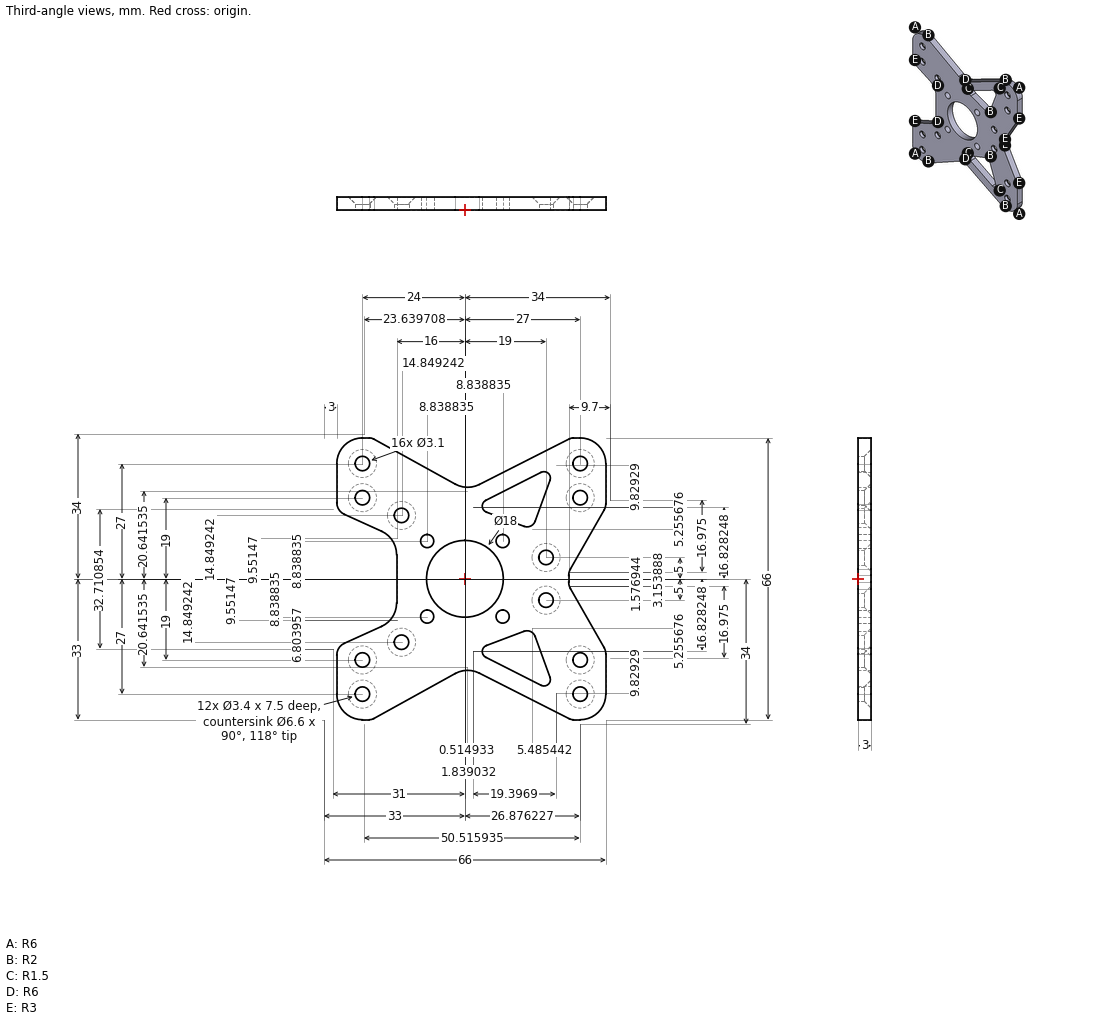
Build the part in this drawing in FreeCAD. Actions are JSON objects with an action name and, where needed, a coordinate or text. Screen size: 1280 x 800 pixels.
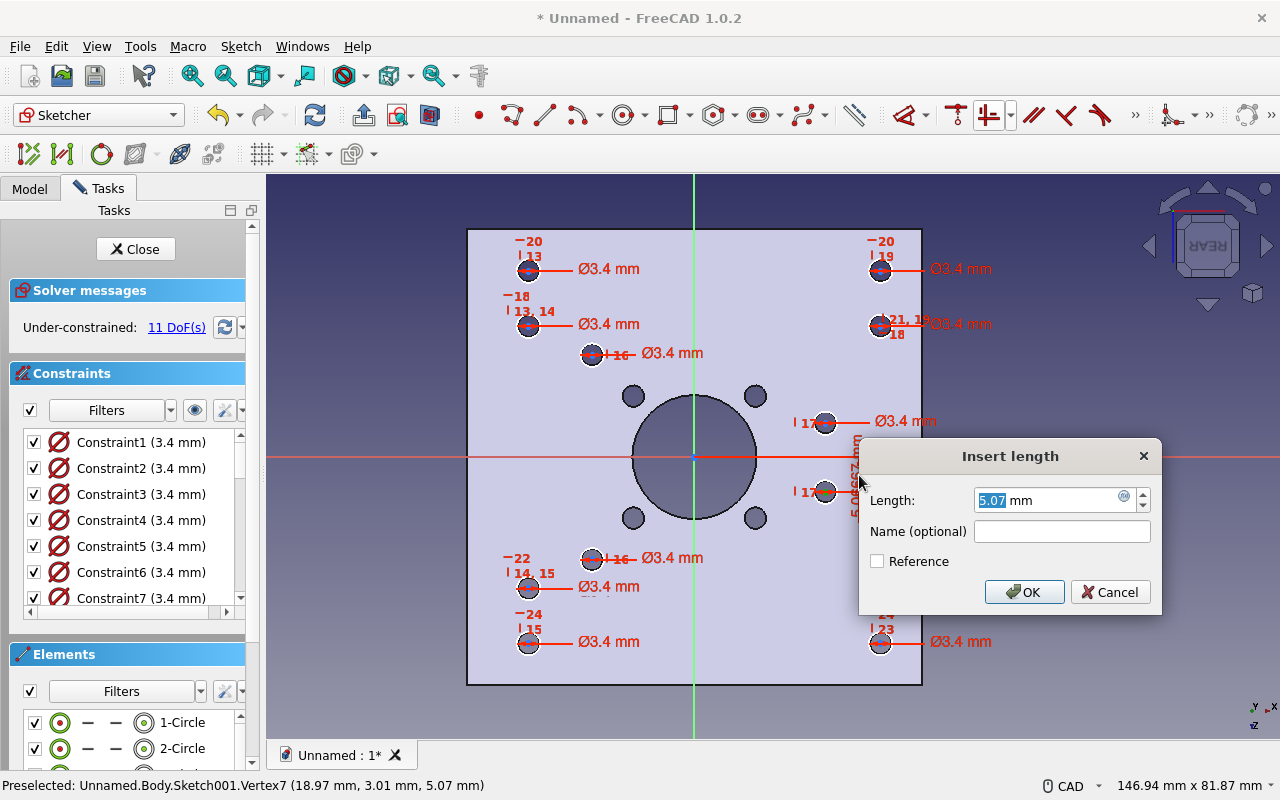
{"action": "type", "text": "5"}
{"action": "key", "text": "Return"}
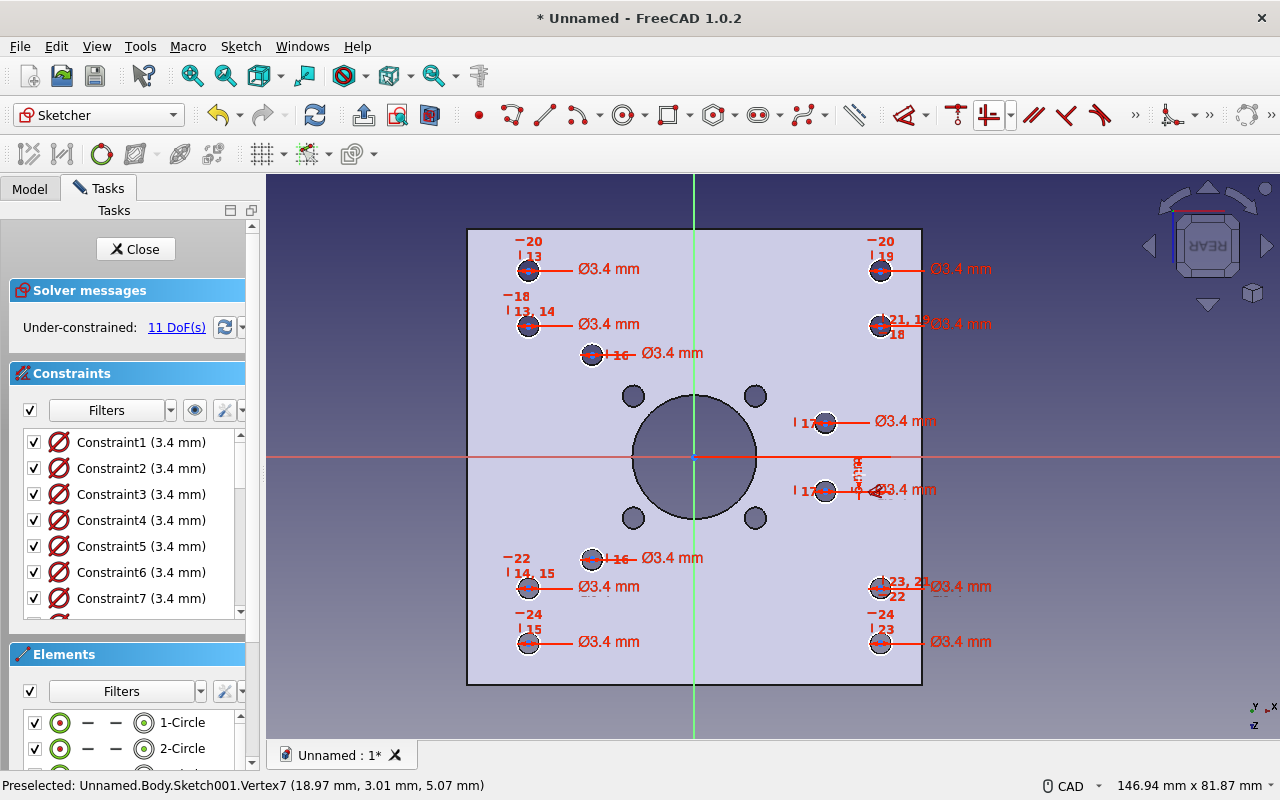
{"action": "left_click", "coordinate": [825, 423]}
{"action": "left_click", "coordinate": [859, 440]}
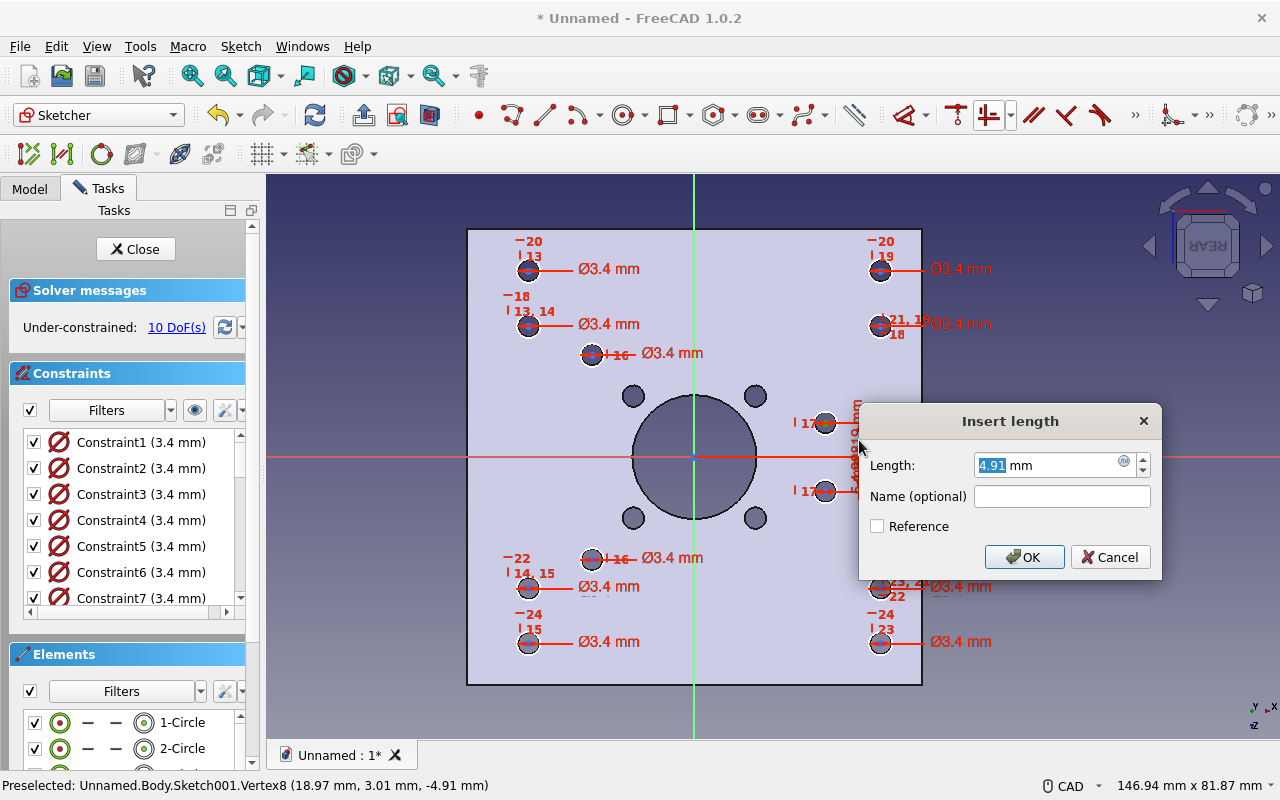
{"action": "type", "text": "5"}
{"action": "key", "text": "Return"}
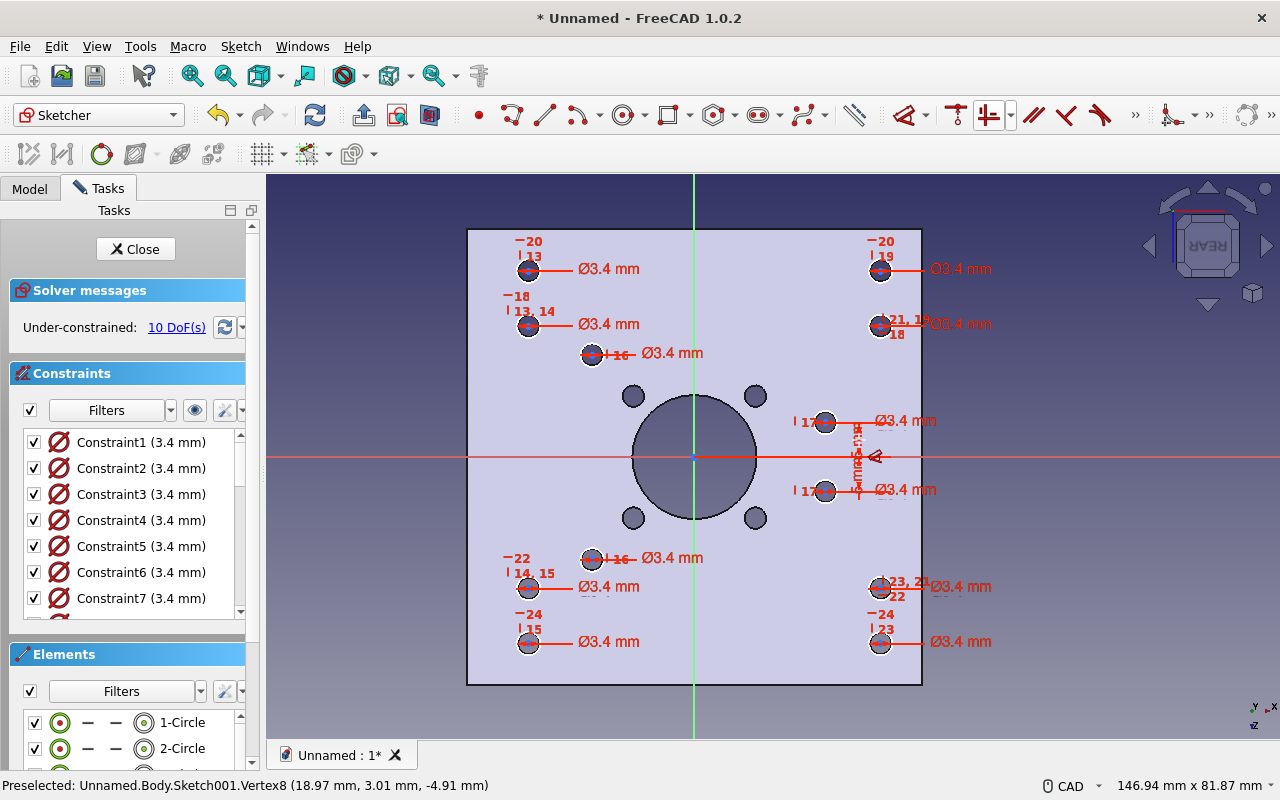
{"action": "left_click", "coordinate": [529, 271]}
{"action": "left_click", "coordinate": [612, 237]}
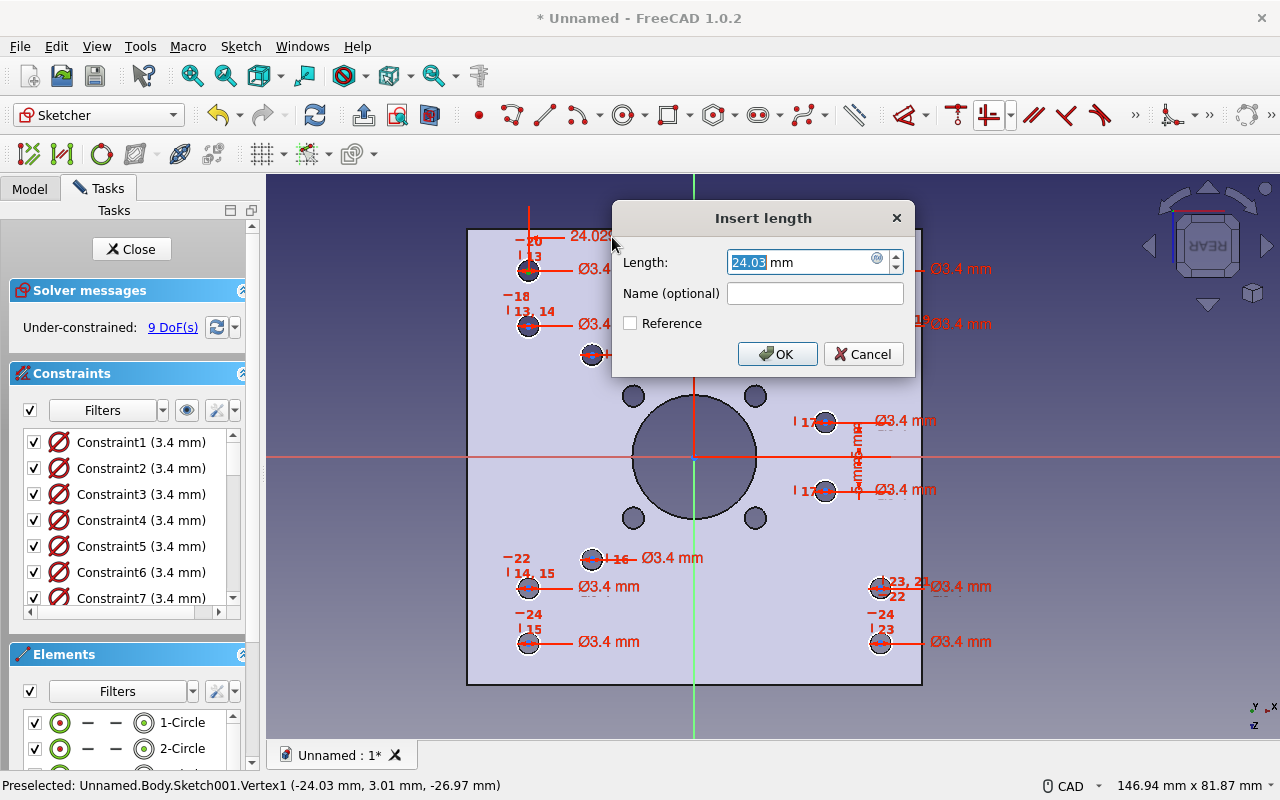
{"action": "type", "text": "24"}
{"action": "key", "text": "Return"}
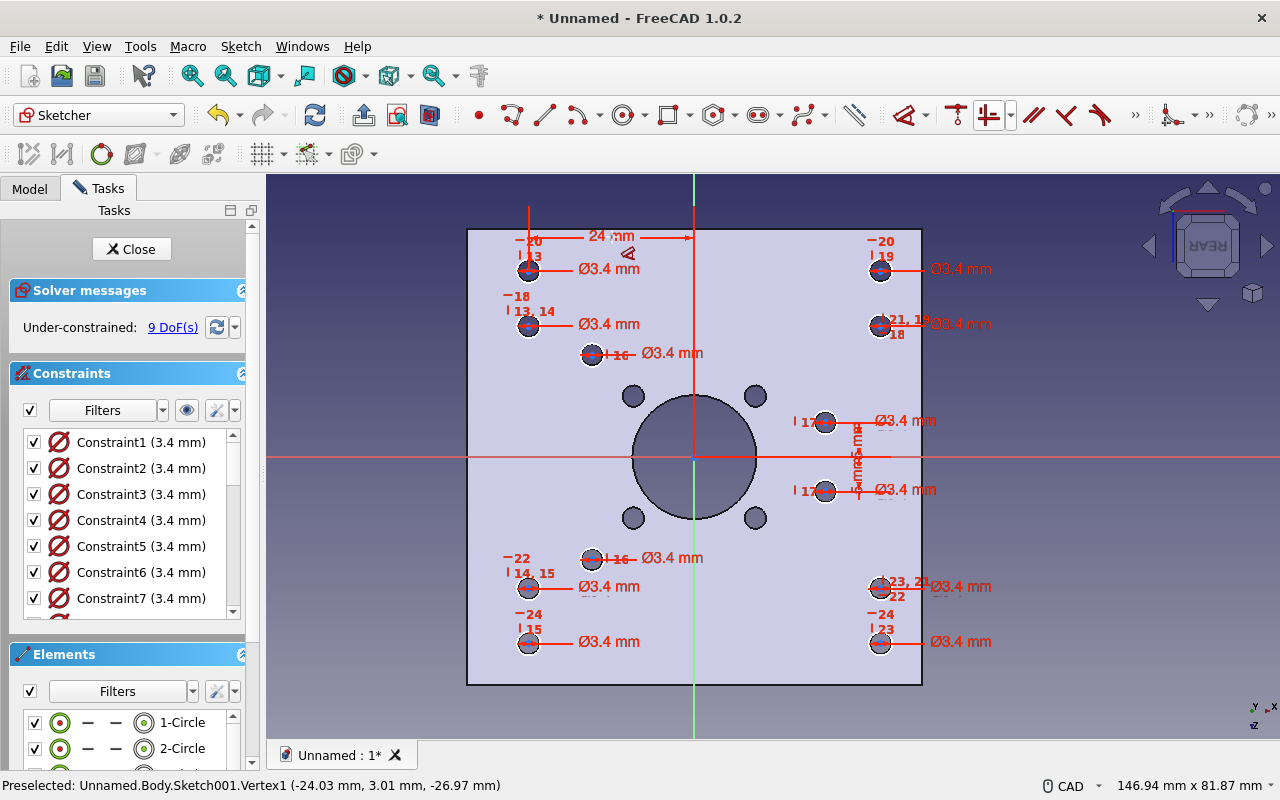
{"action": "left_click", "coordinate": [529, 271]}
{"action": "left_click", "coordinate": [495, 364]}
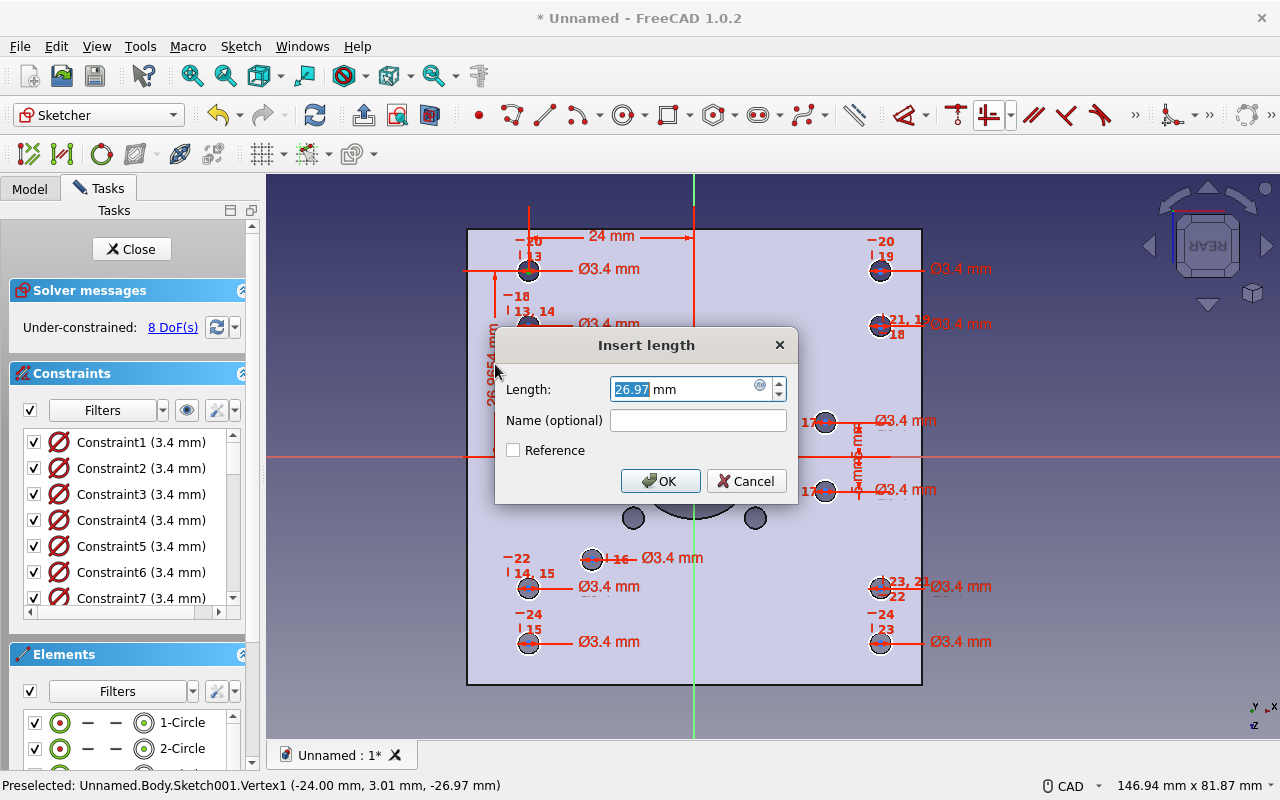
{"action": "type", "text": "27"}
{"action": "key", "text": "Return"}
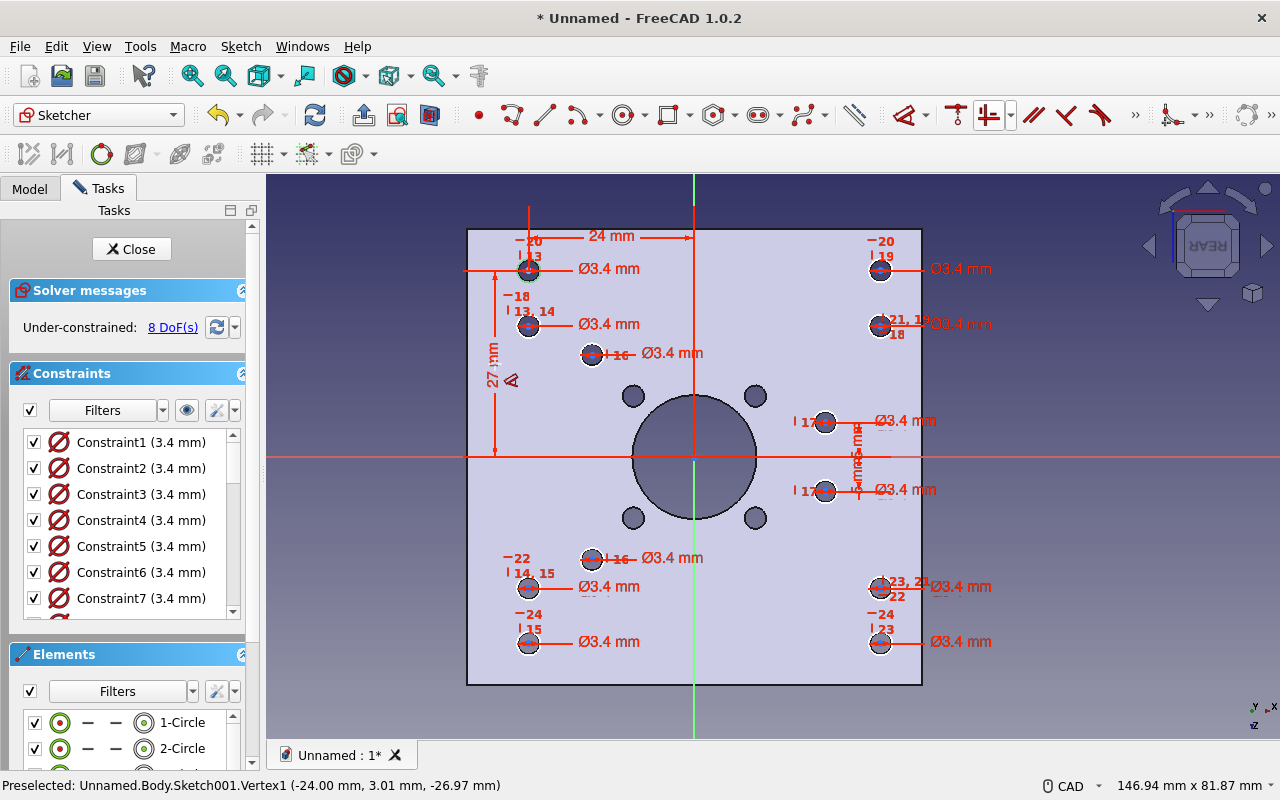
{"action": "left_click", "coordinate": [529, 326]}
{"action": "left_click", "coordinate": [495, 392]}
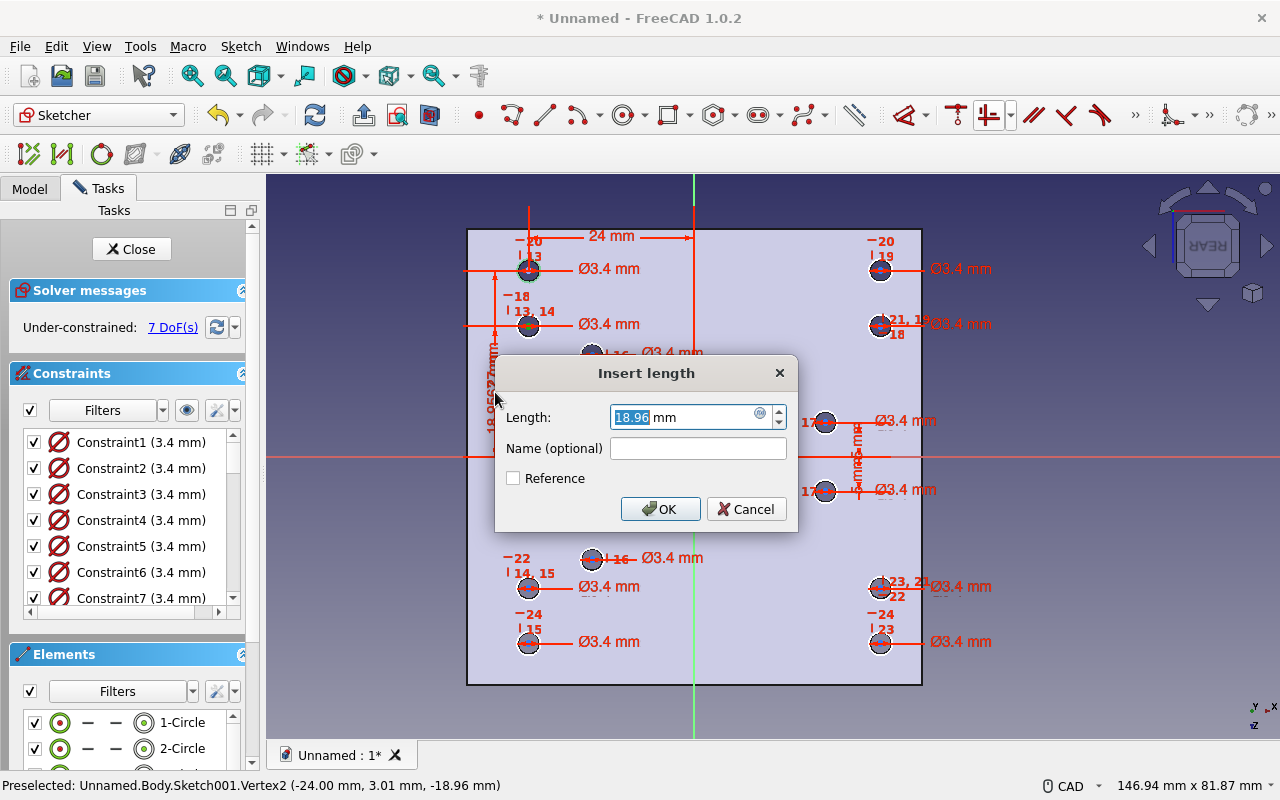
{"action": "type", "text": "19"}
{"action": "key", "text": "Return"}